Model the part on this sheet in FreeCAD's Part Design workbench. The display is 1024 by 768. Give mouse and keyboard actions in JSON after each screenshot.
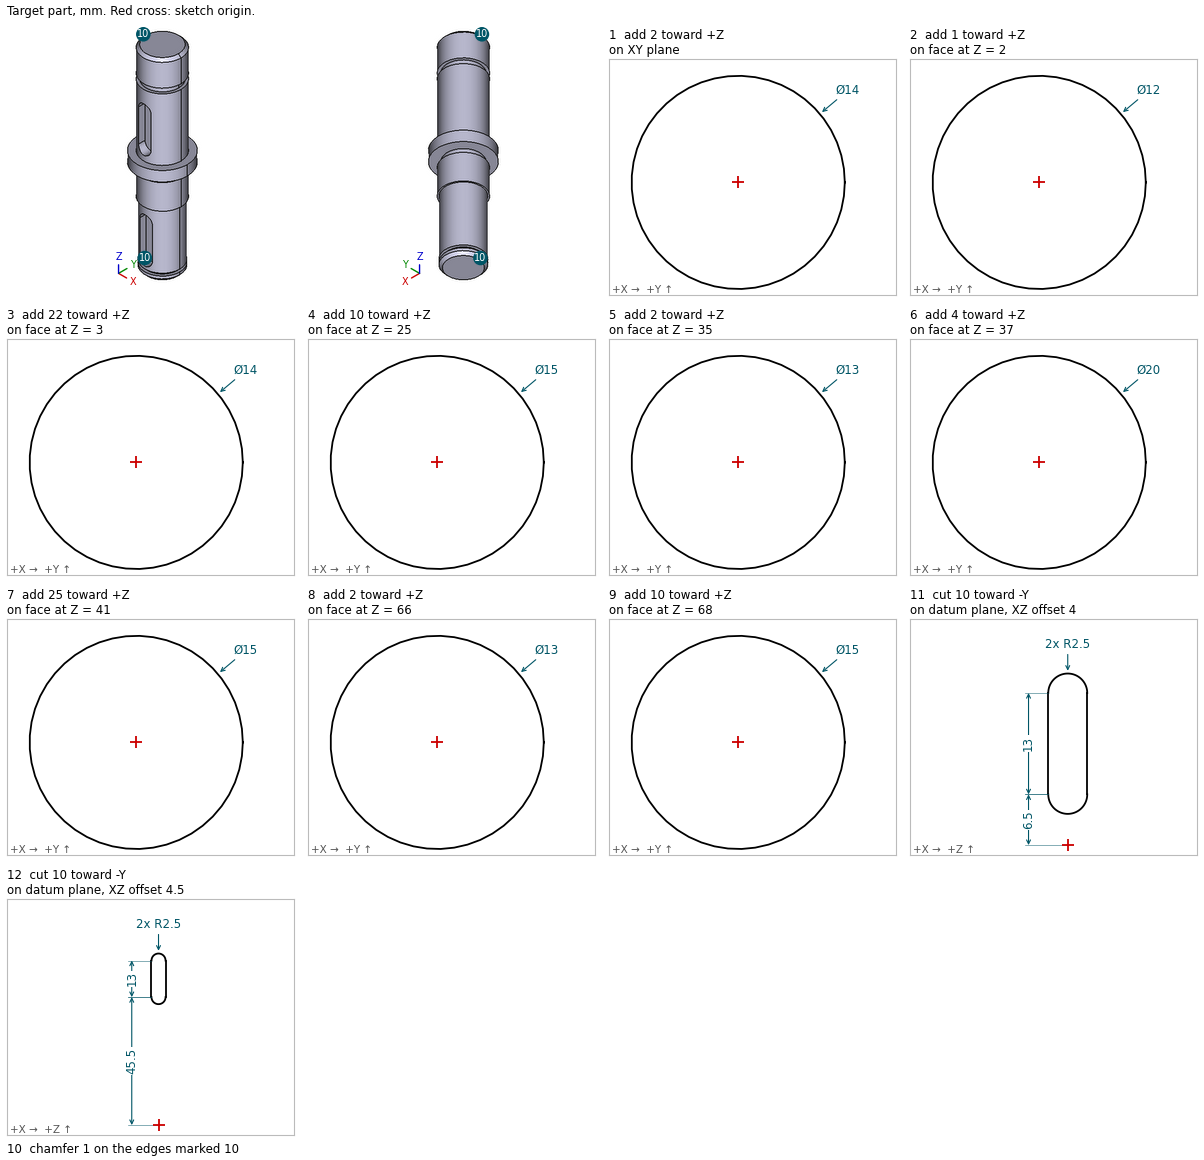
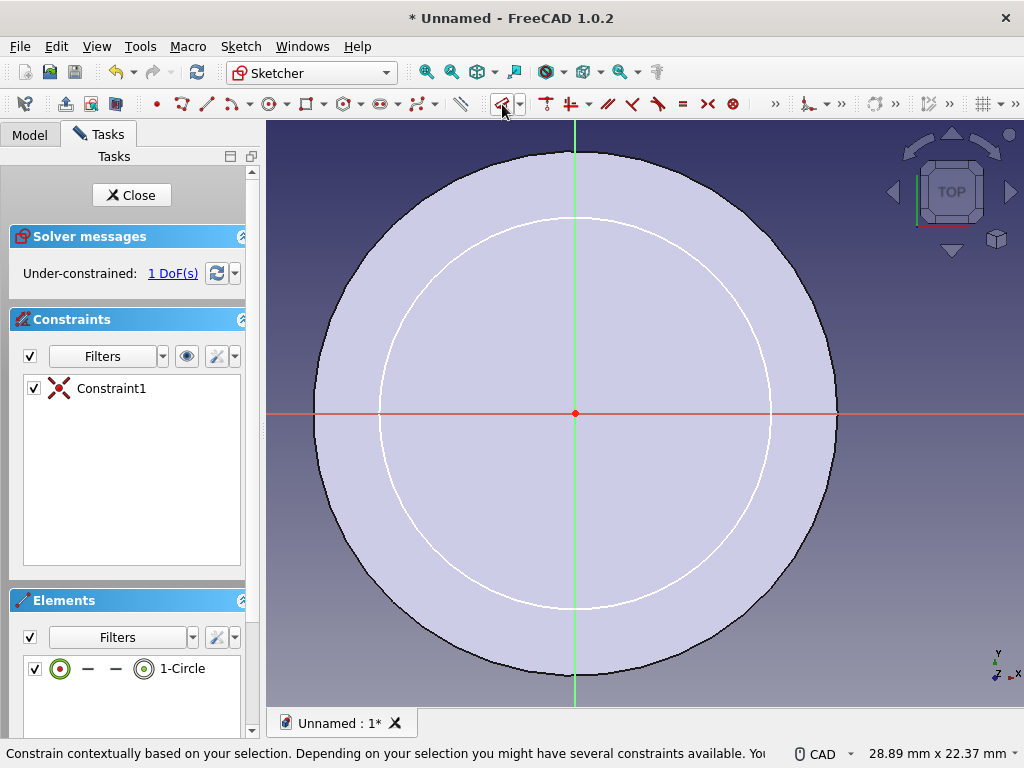
{"action": "left_click", "coordinate": [713, 274]}
{"action": "left_click", "coordinate": [735, 251]}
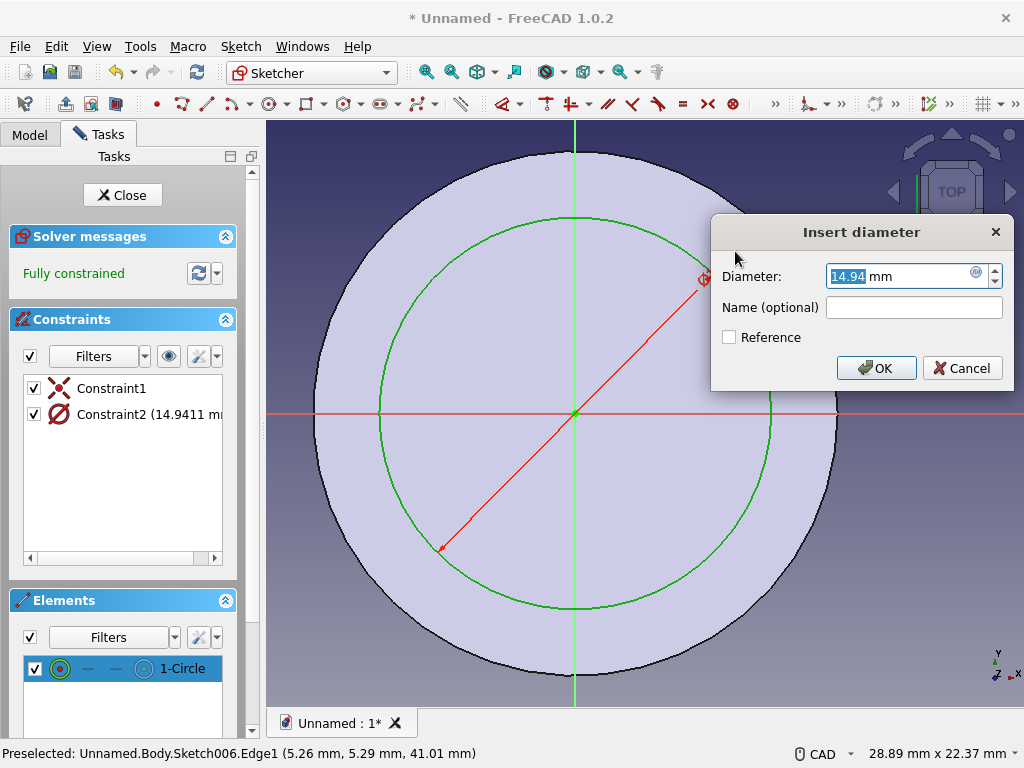
{"action": "type", "text": "15"}
{"action": "key", "text": "Return"}
{"action": "key", "text": "Escape"}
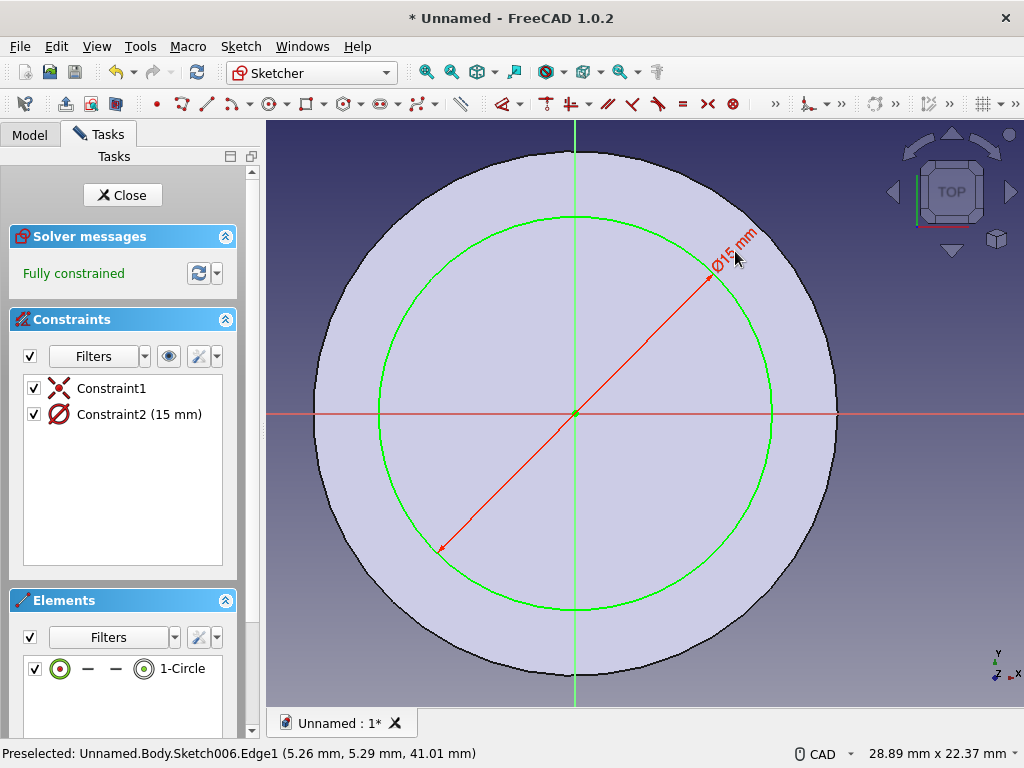
{"action": "left_click", "coordinate": [123, 195]}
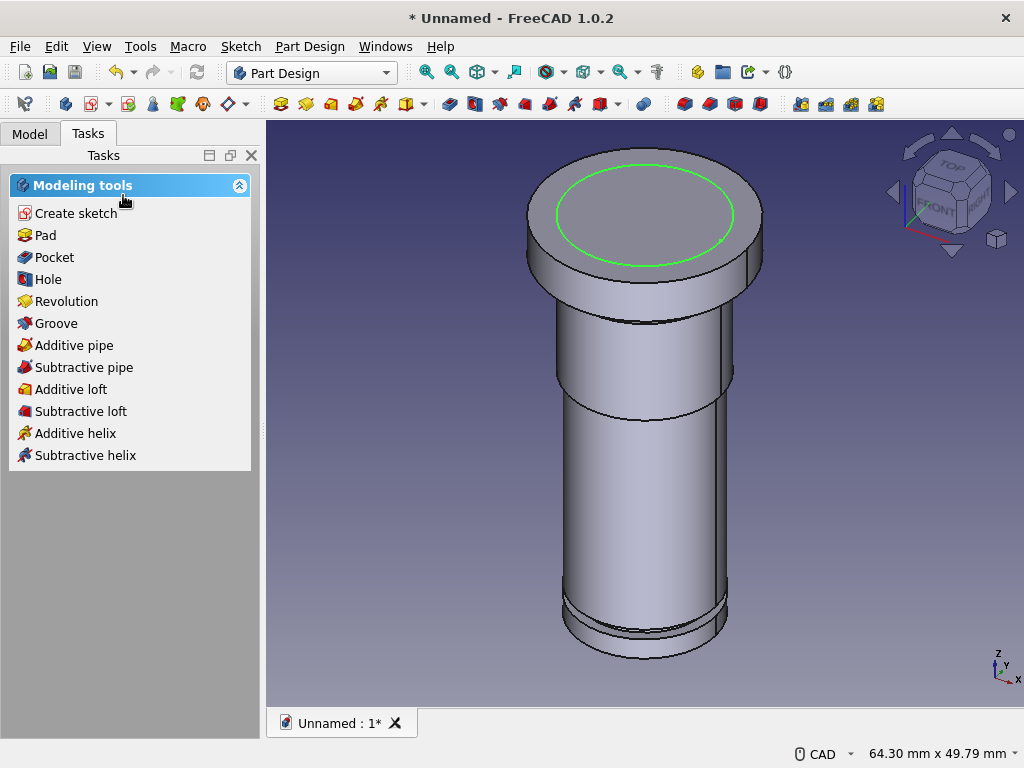
{"action": "left_click", "coordinate": [281, 104]}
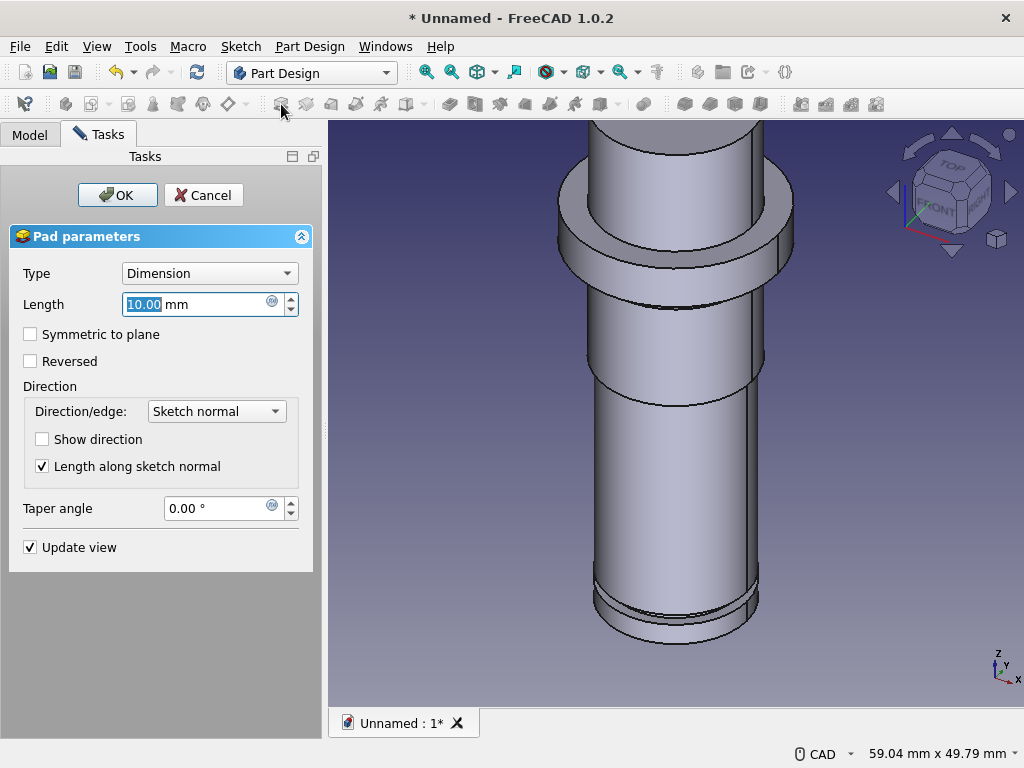
{"action": "type", "text": "25"}
{"action": "key", "text": "Tab"}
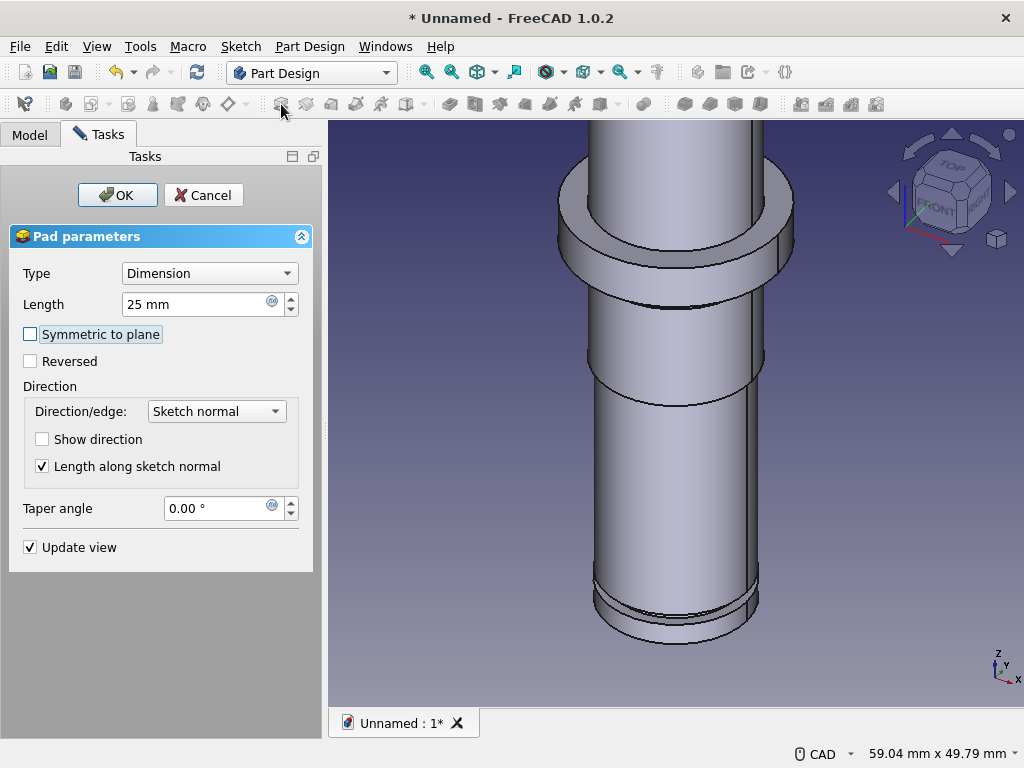
{"action": "left_click", "coordinate": [118, 195]}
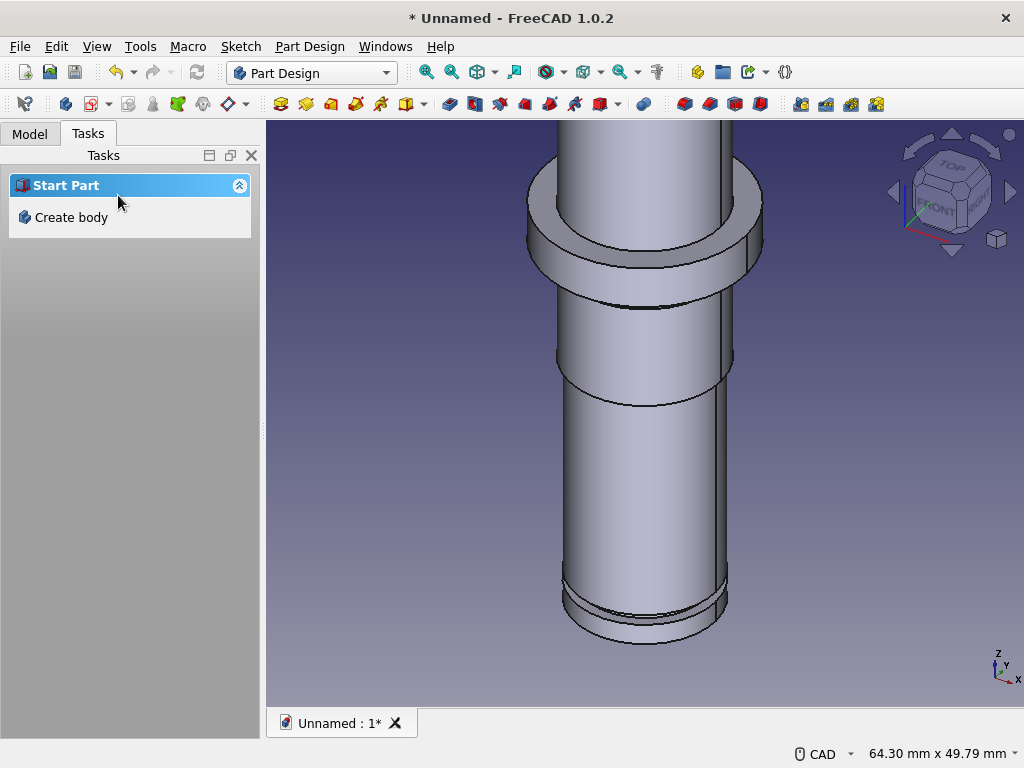
{"action": "key", "text": "v f"}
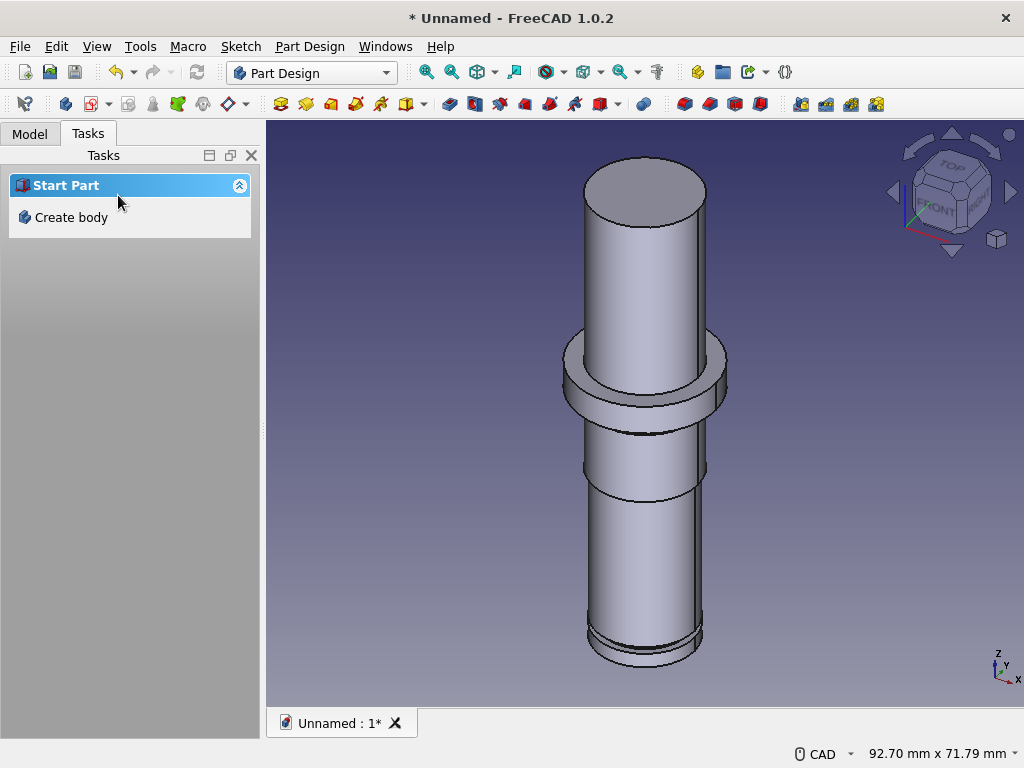
{"action": "left_click", "coordinate": [645, 191]}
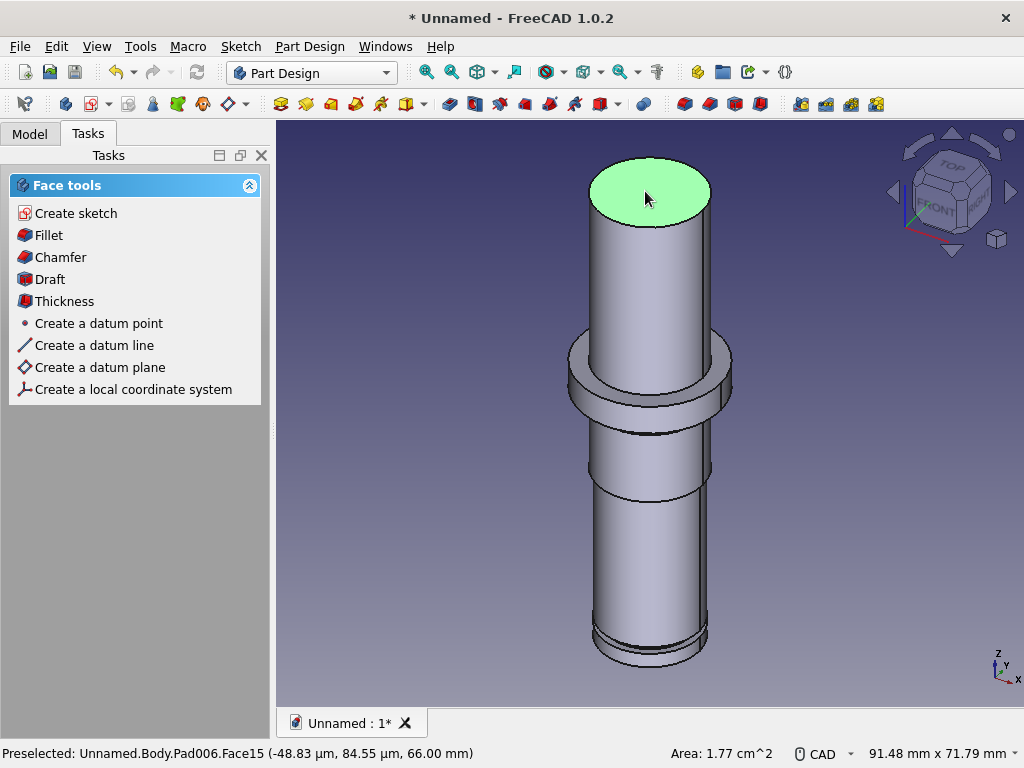
{"action": "left_click", "coordinate": [90, 104]}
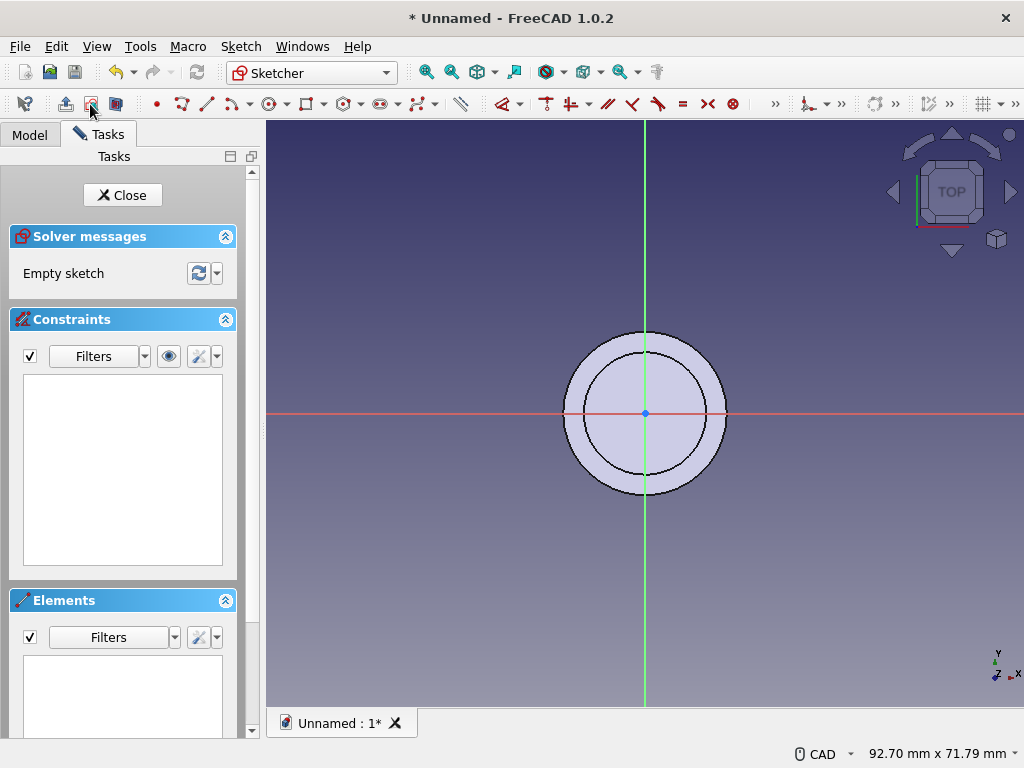
{"action": "scroll", "coordinate": [675, 414], "scroll_direction": "up", "scroll_amount": 6}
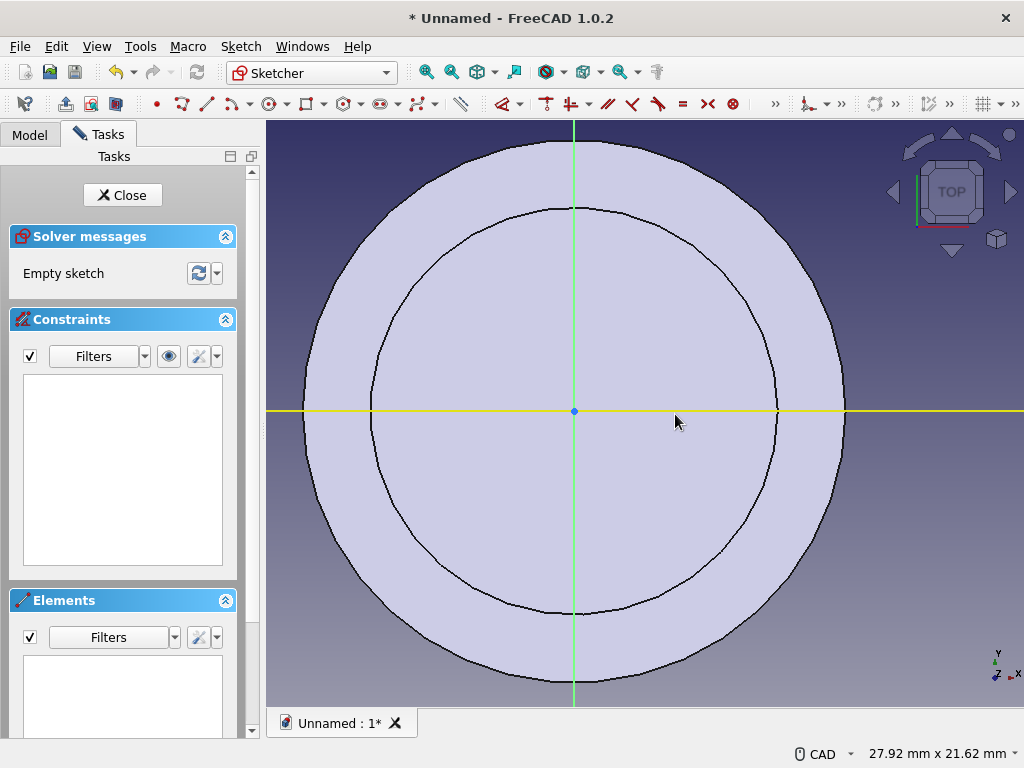
{"action": "left_click", "coordinate": [268, 104]}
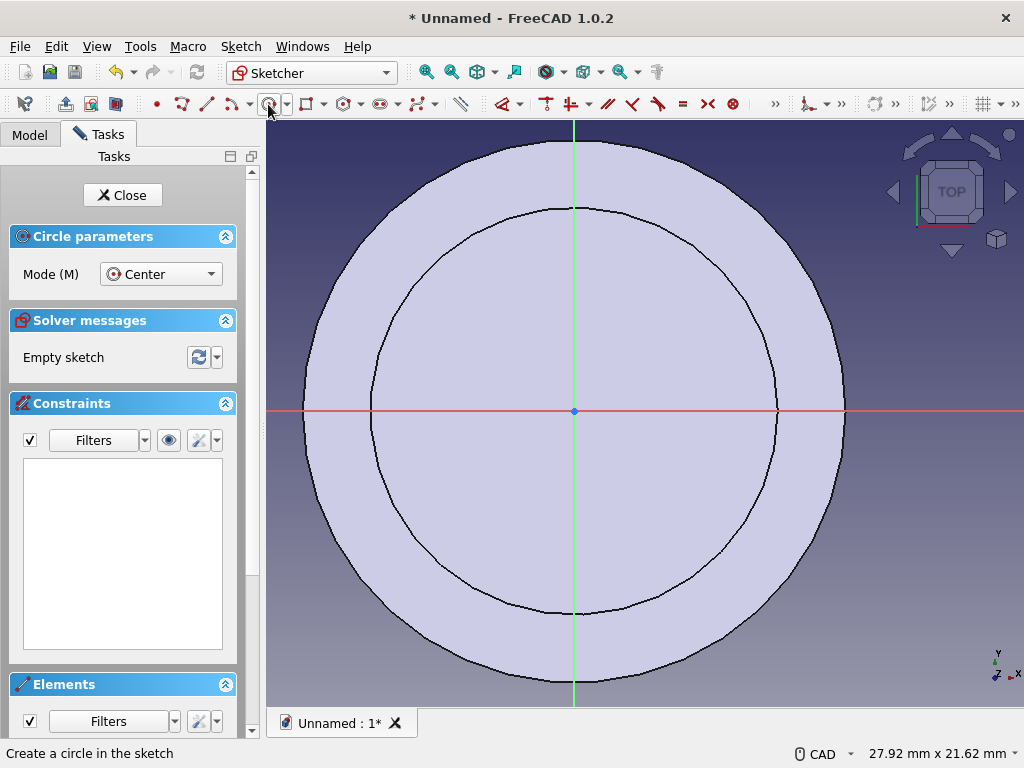
{"action": "left_click", "coordinate": [574, 411]}
{"action": "left_click", "coordinate": [699, 286]}
{"action": "key", "text": "Escape"}